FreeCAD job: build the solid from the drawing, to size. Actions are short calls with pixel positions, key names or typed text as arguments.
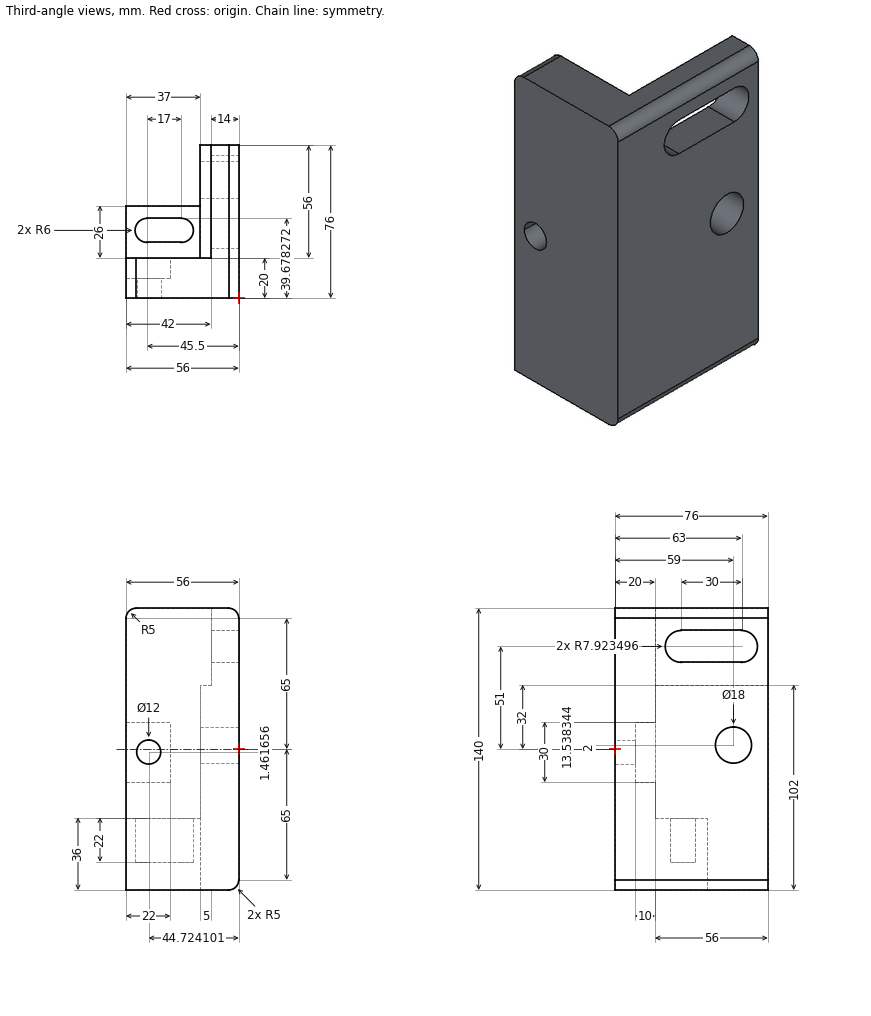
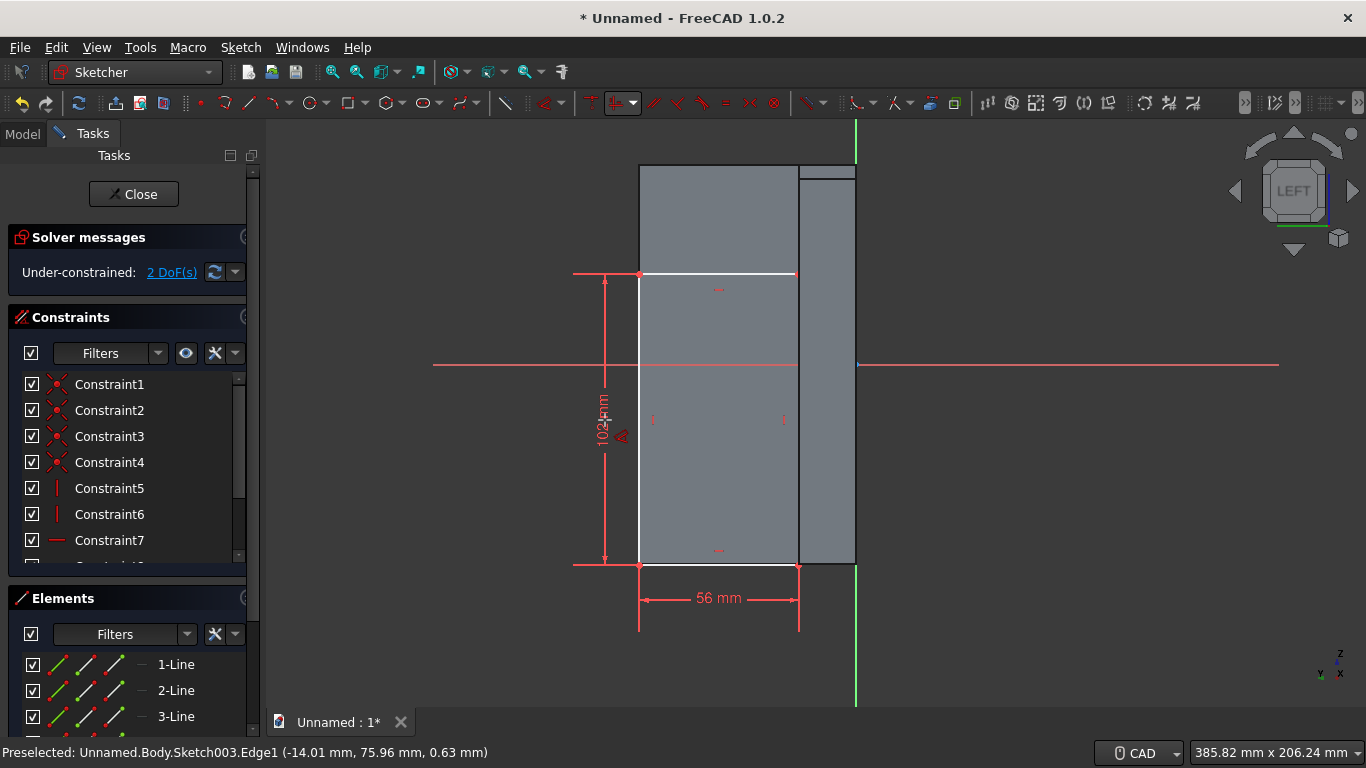
click(639, 274)
click(748, 240)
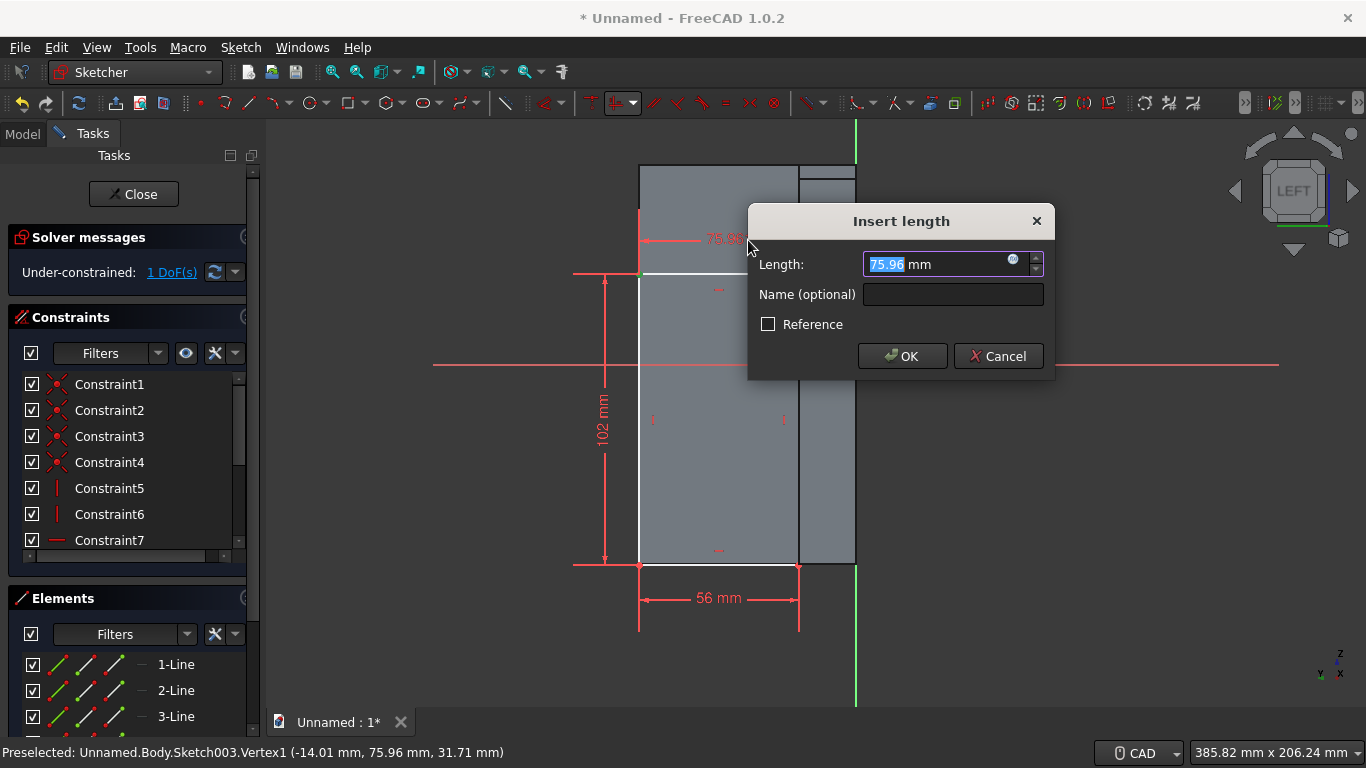
text(76)
key(Return)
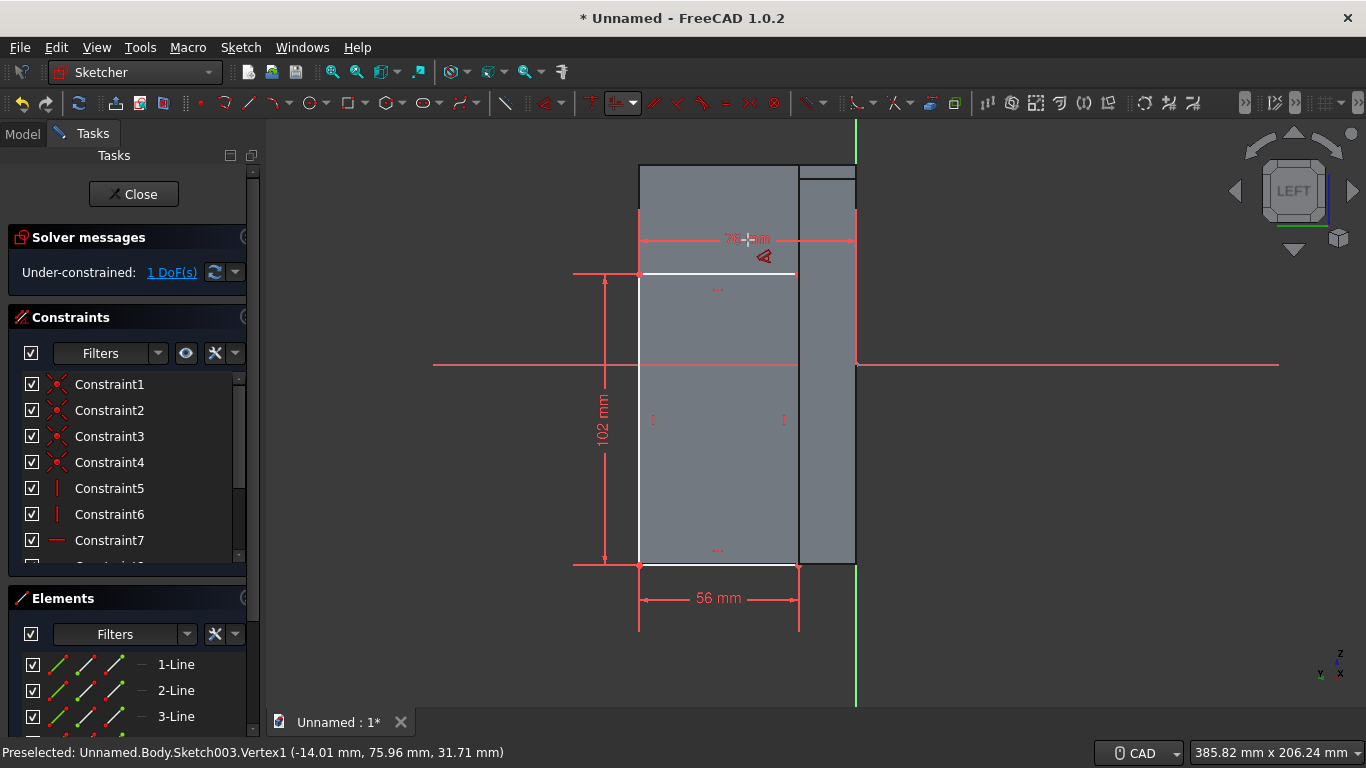
click(639, 274)
click(890, 320)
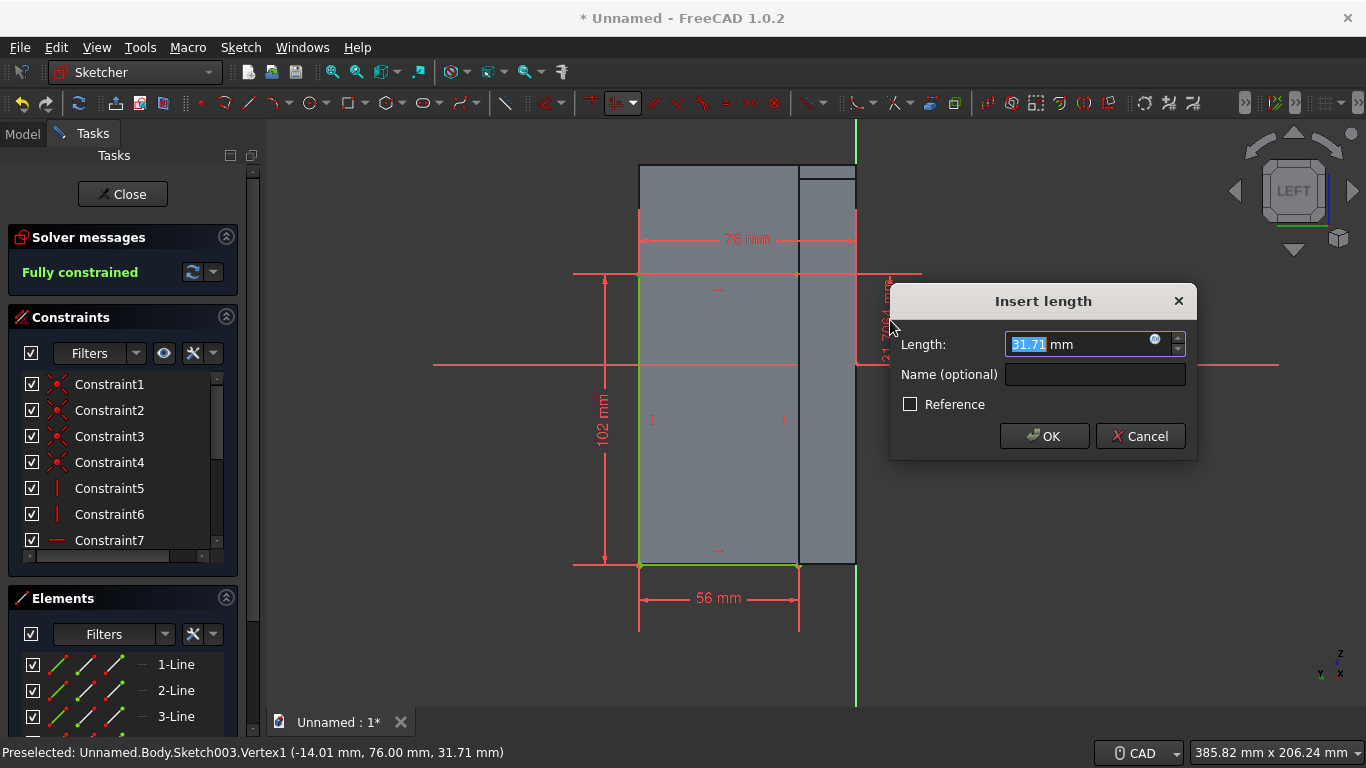
text(32)
key(Return)
key(Escape)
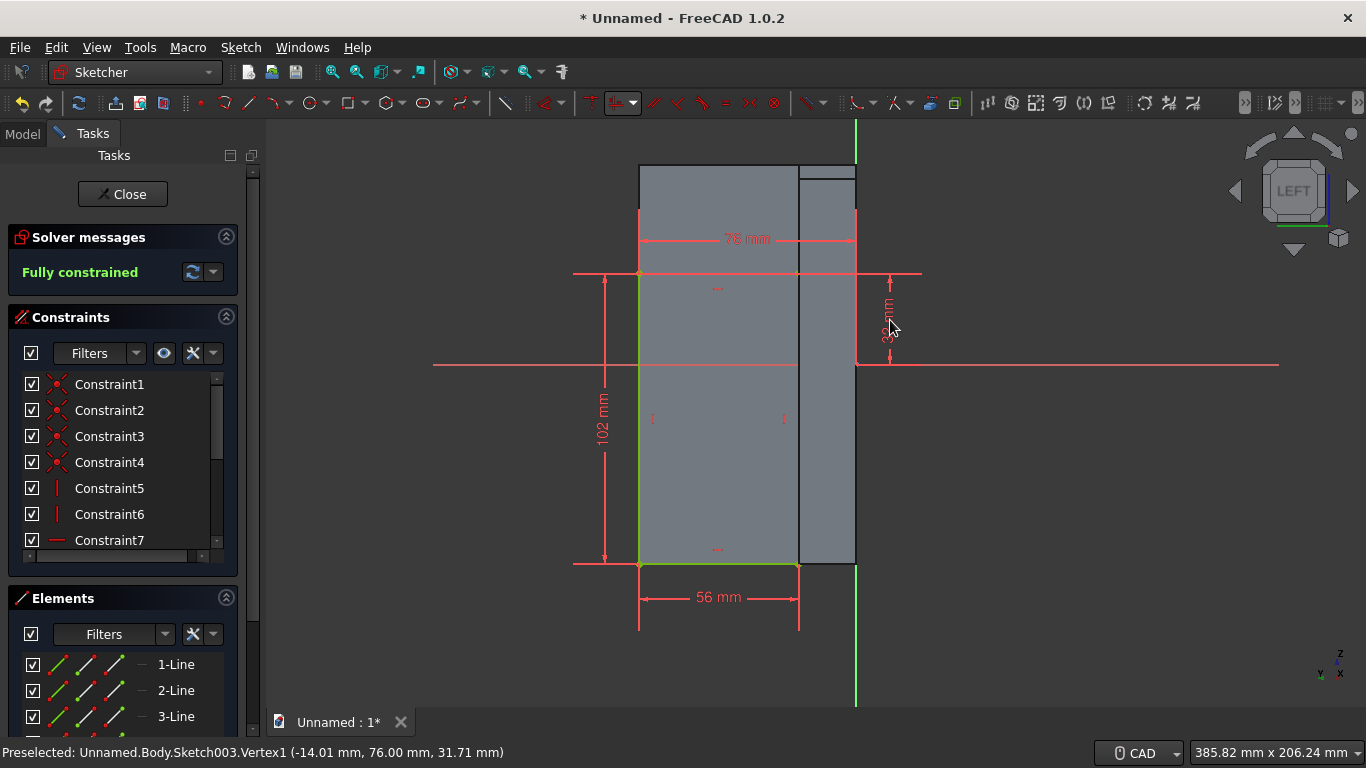
click(123, 194)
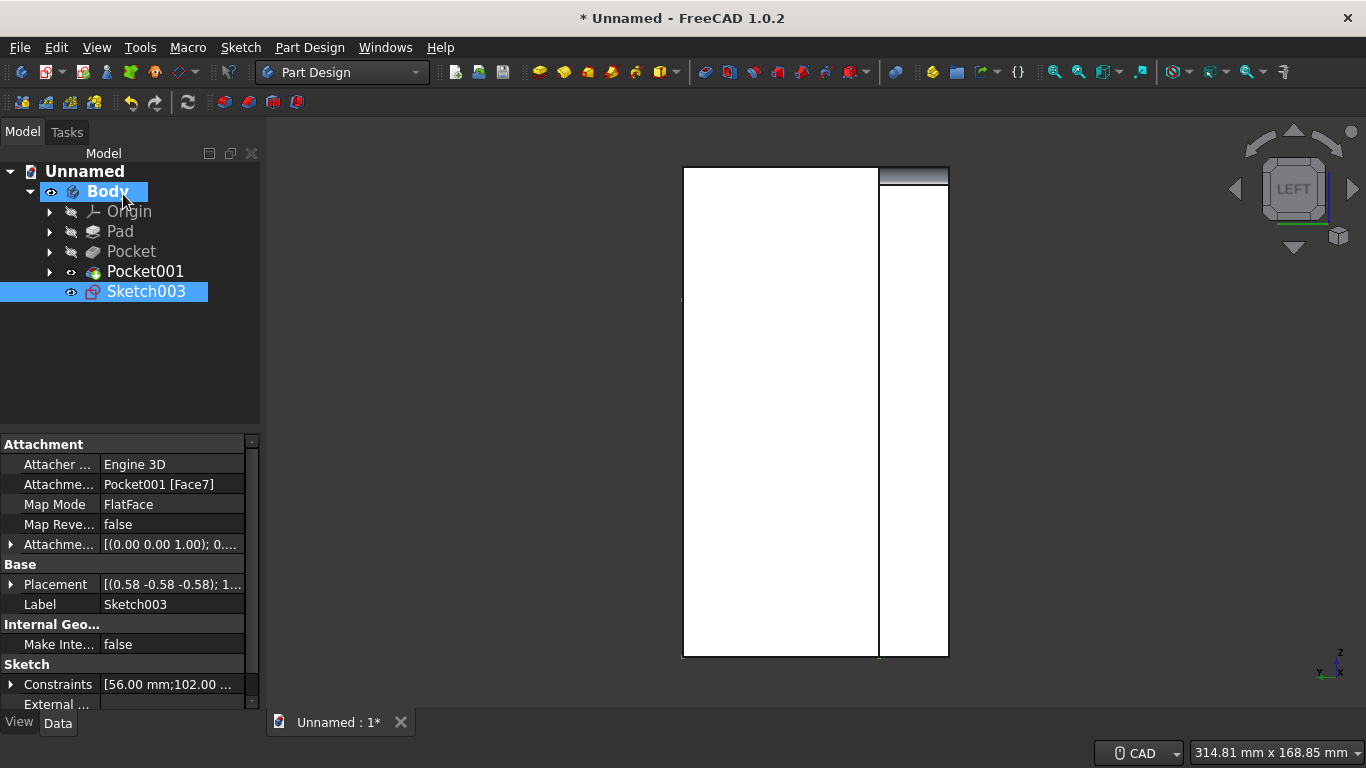
click(540, 72)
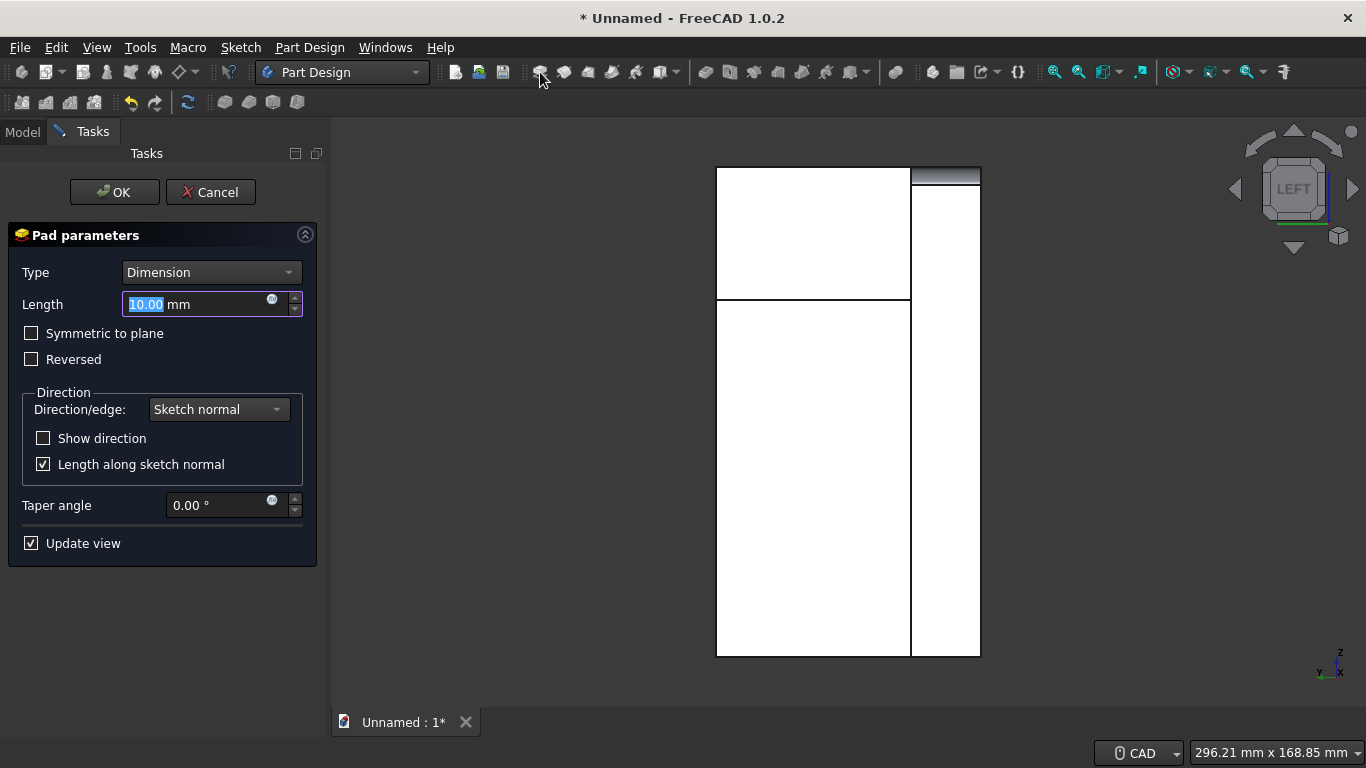
text(5)
key(Tab)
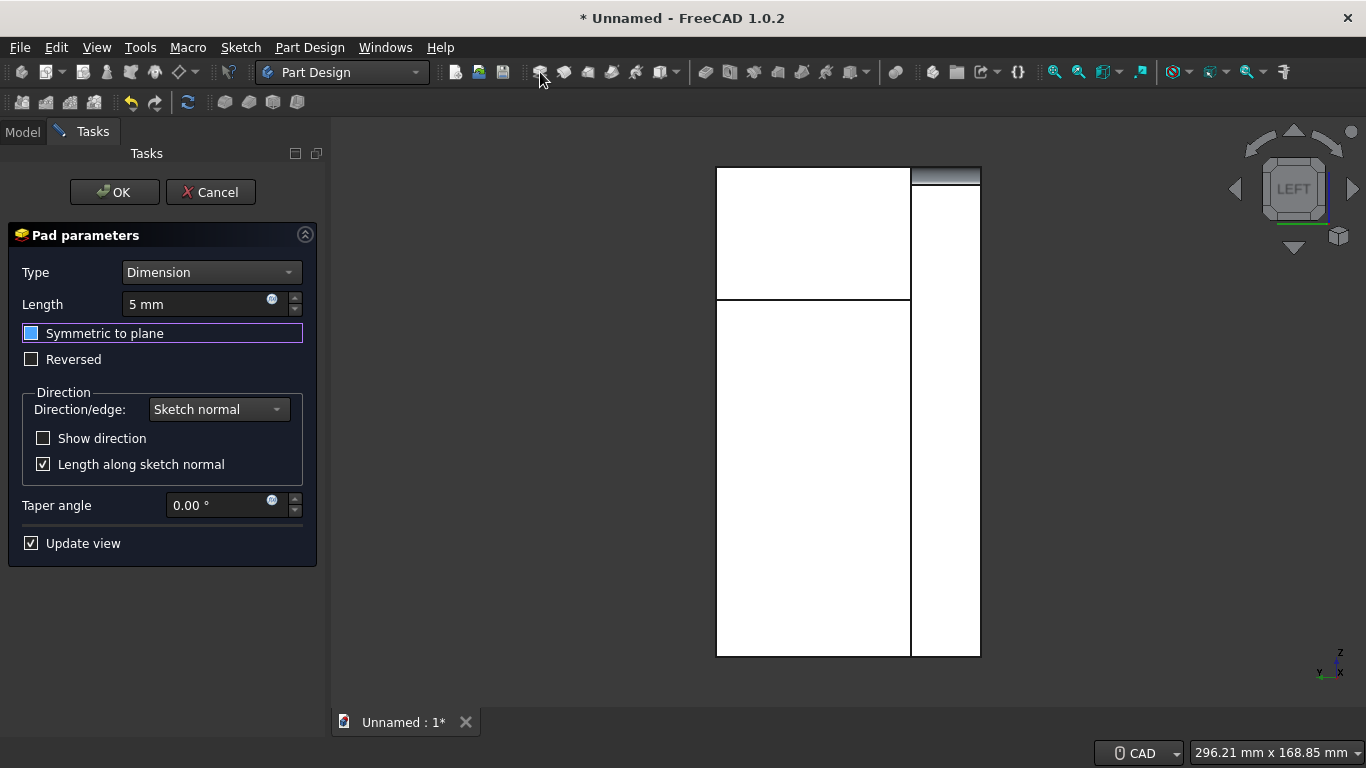
click(115, 192)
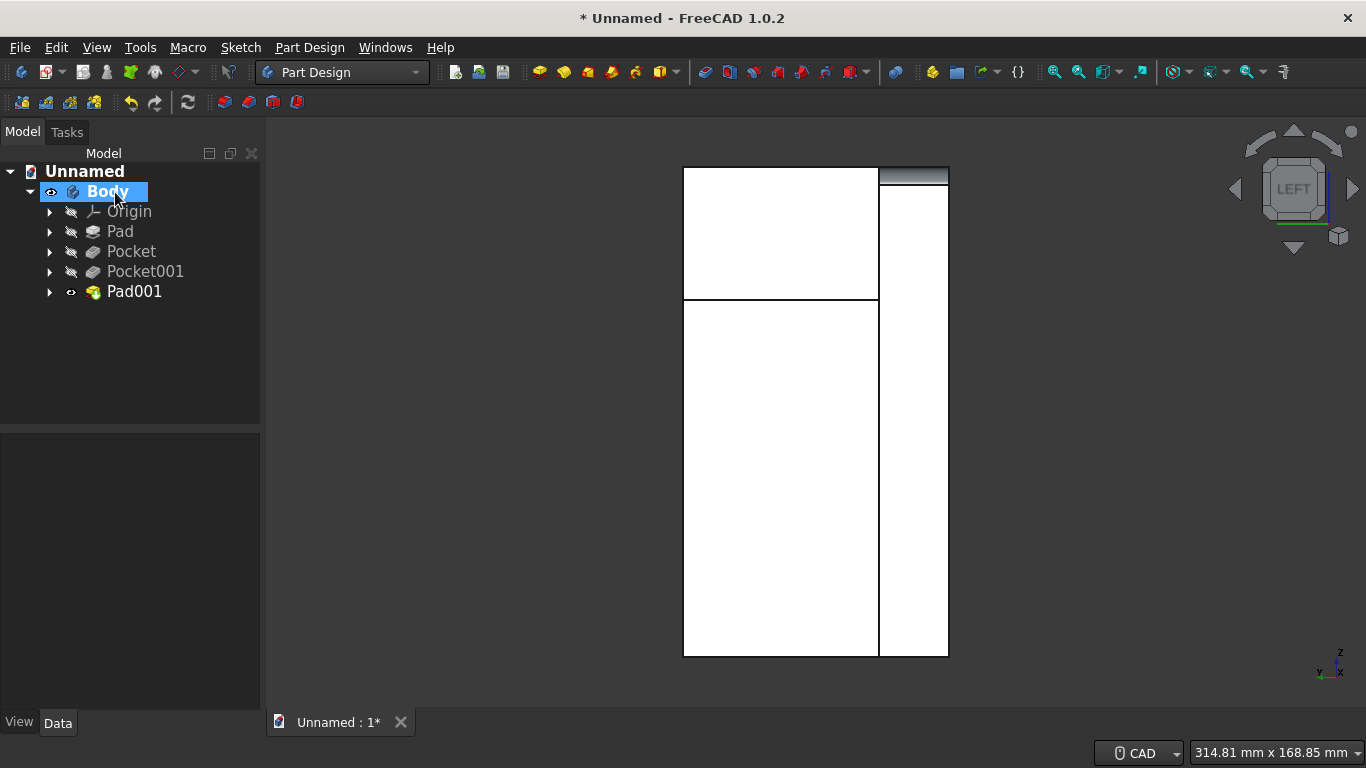
click(753, 233)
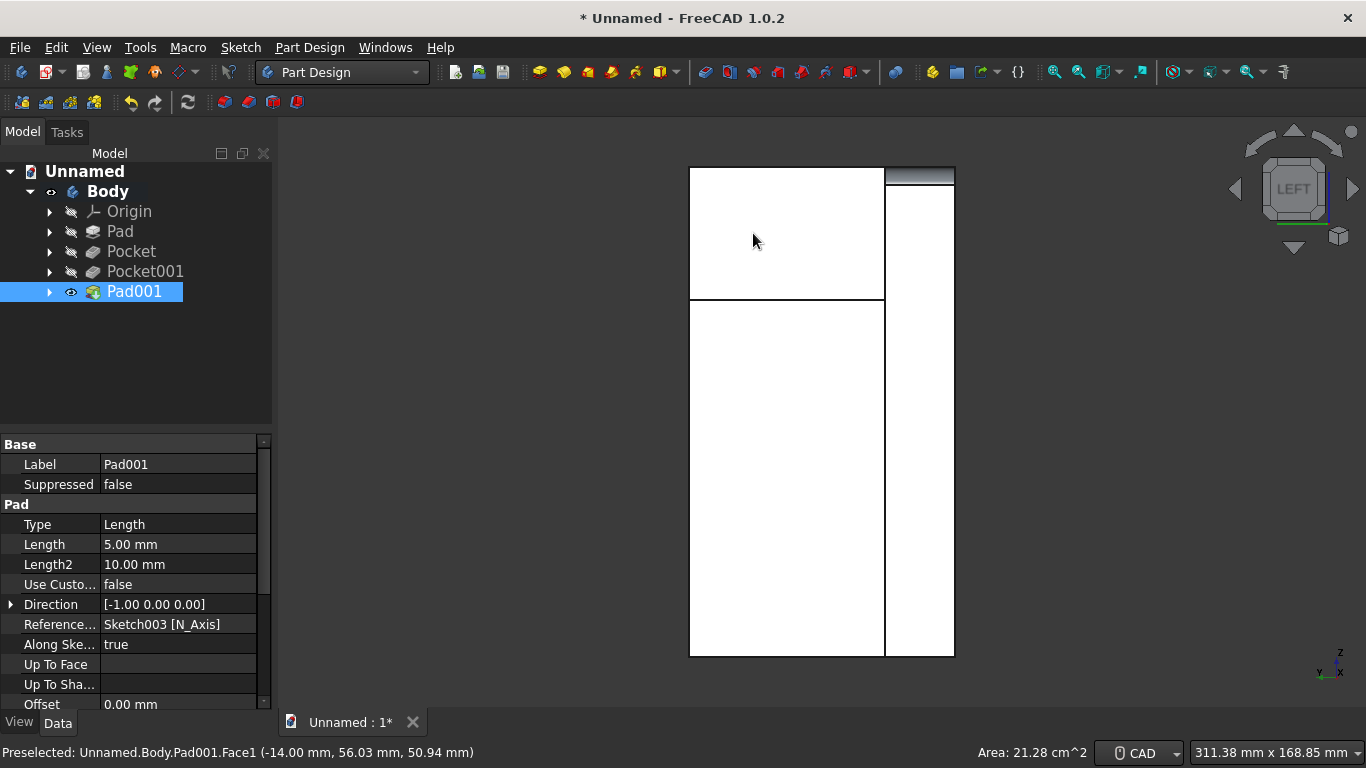
click(46, 72)